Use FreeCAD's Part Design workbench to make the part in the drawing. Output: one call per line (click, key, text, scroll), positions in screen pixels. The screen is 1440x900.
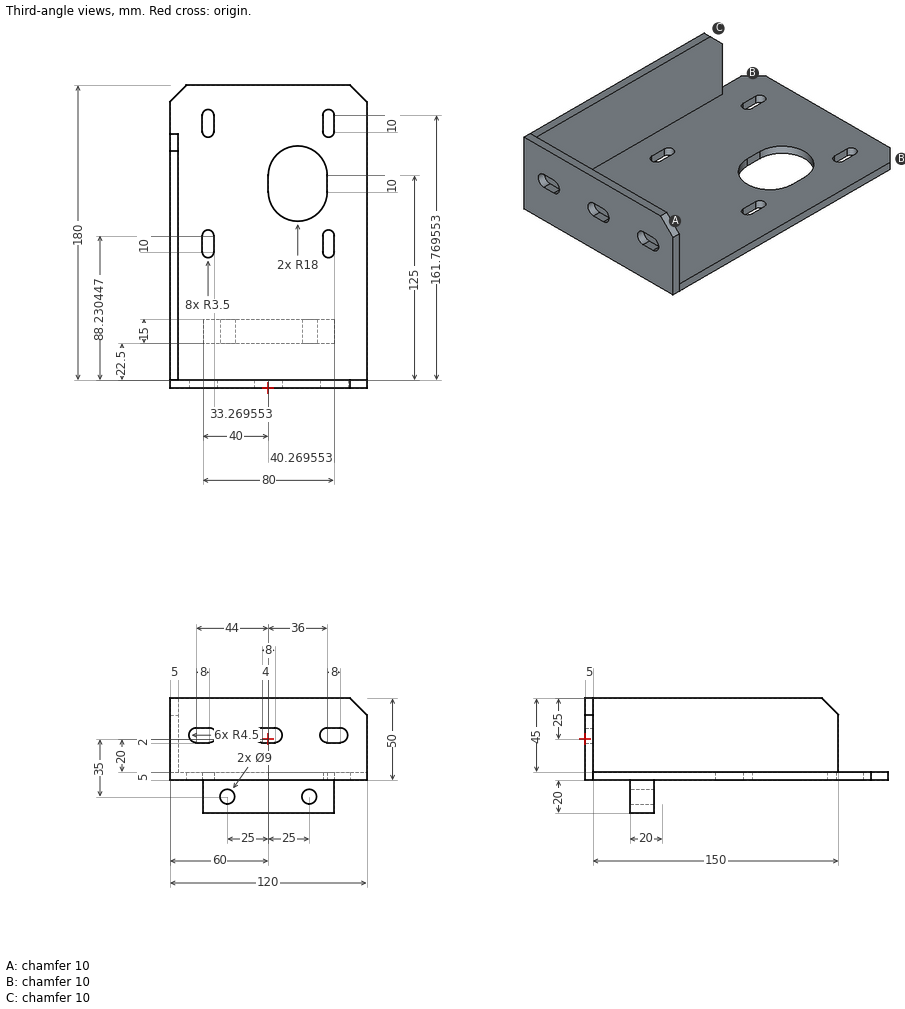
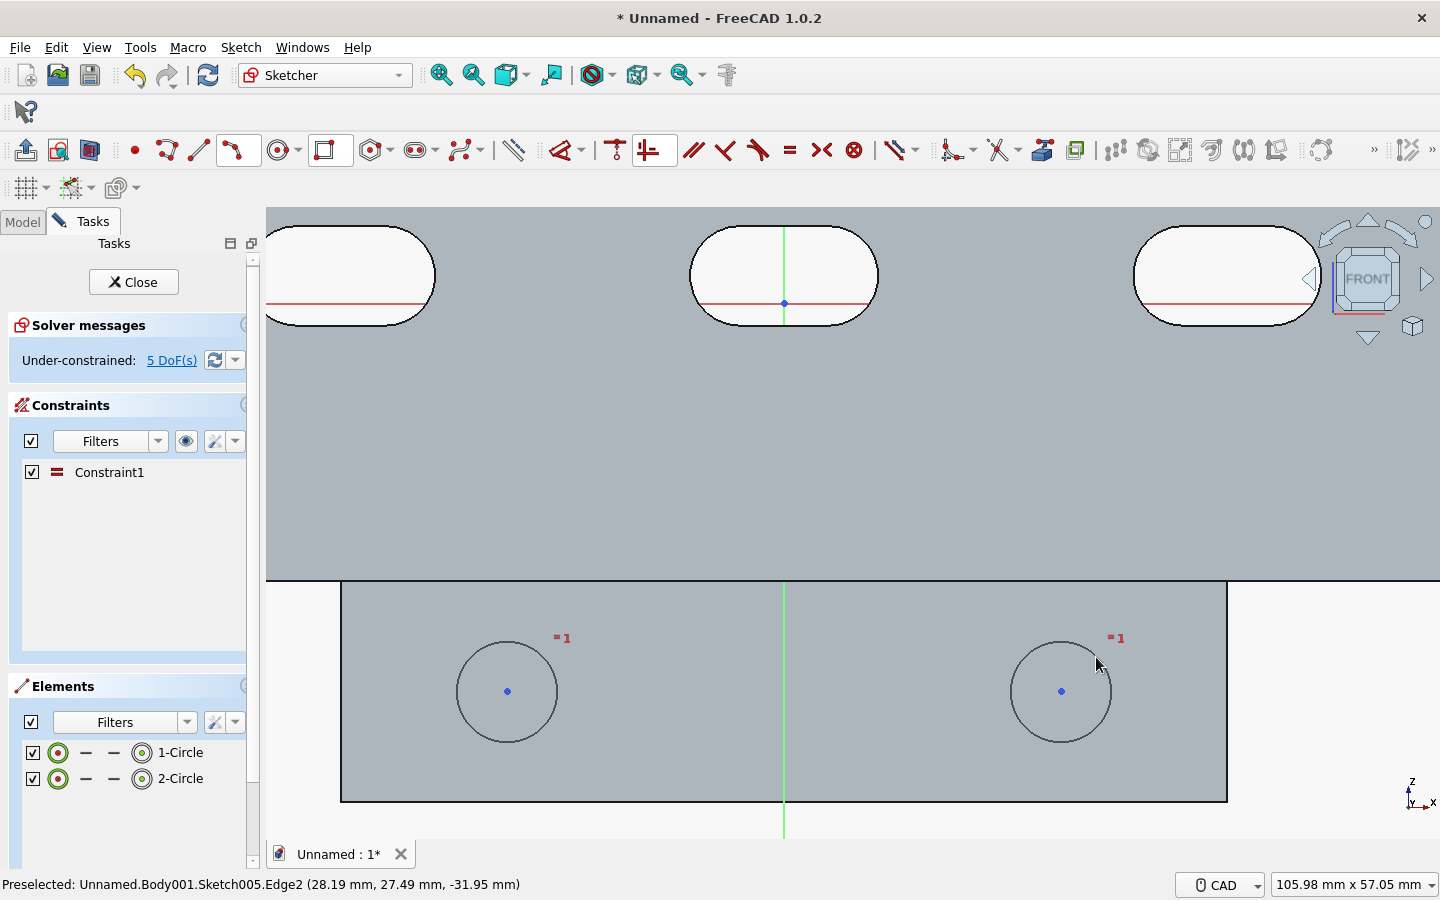
click(560, 150)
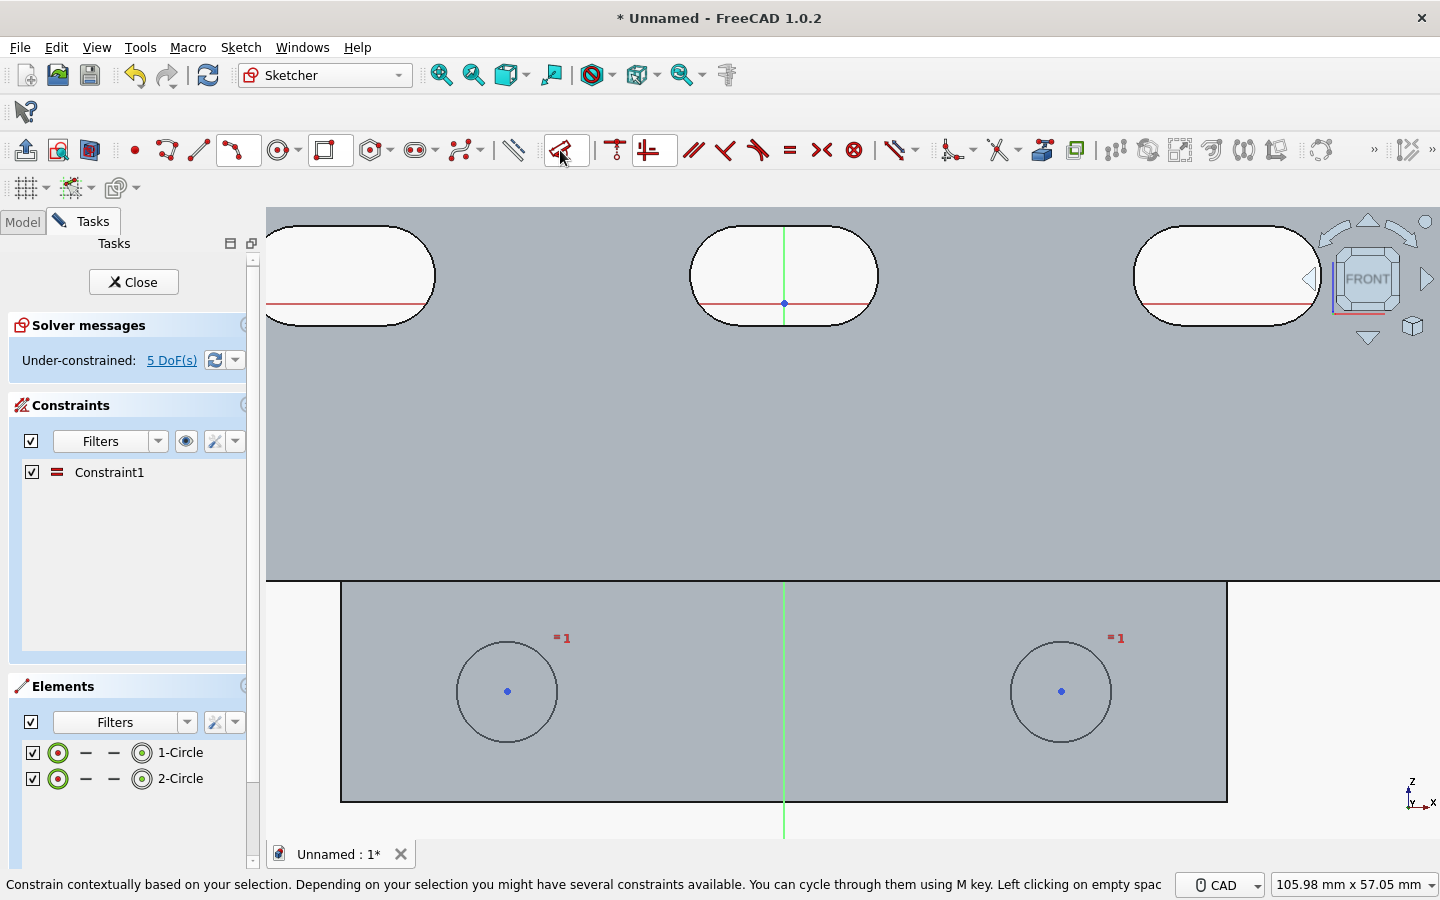
click(542, 656)
click(564, 633)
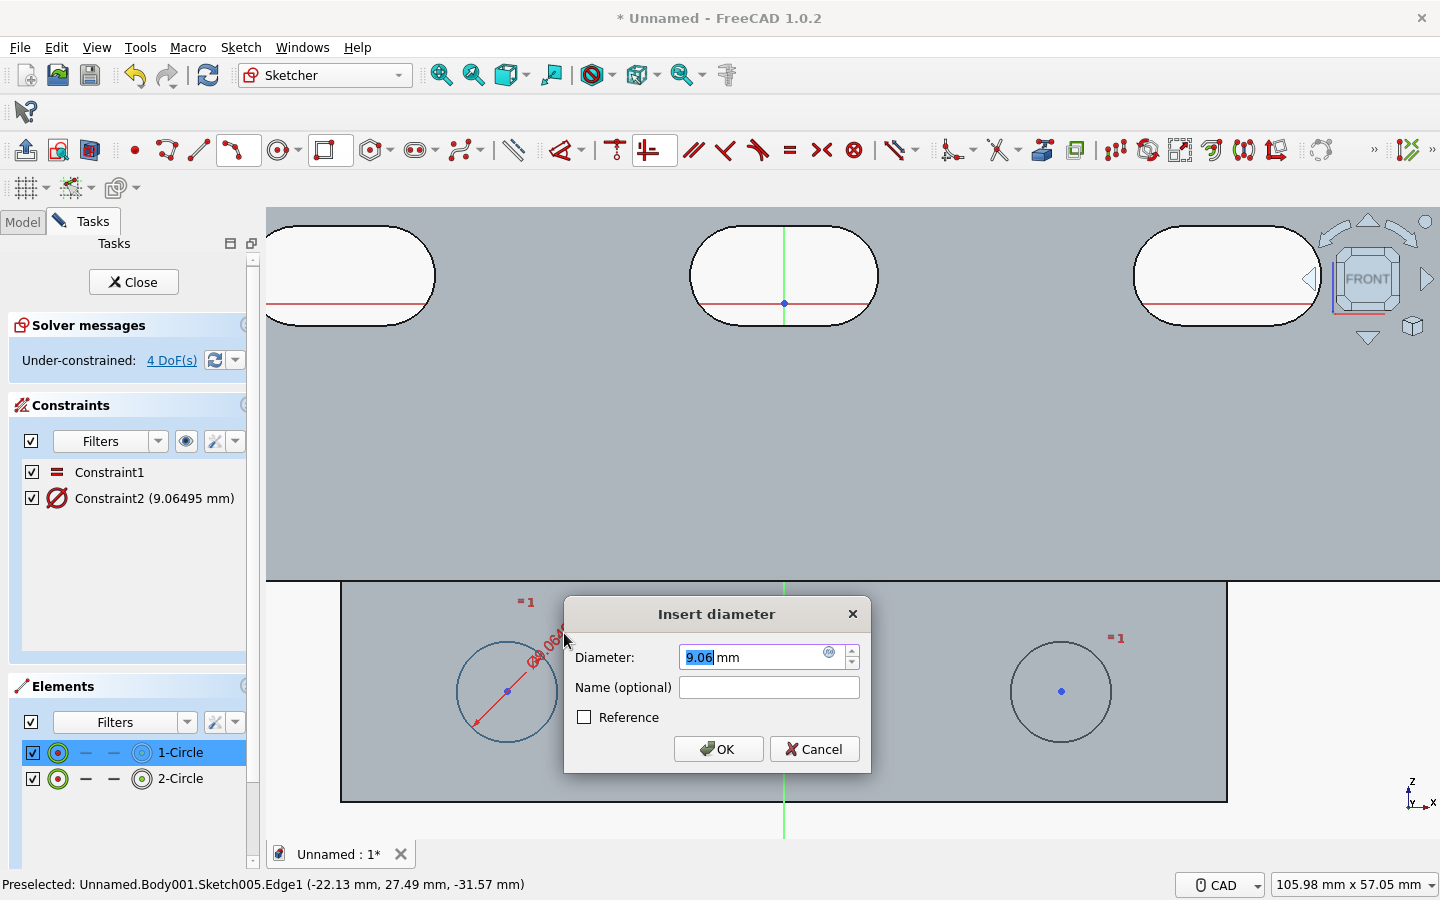
text(9)
key(Return)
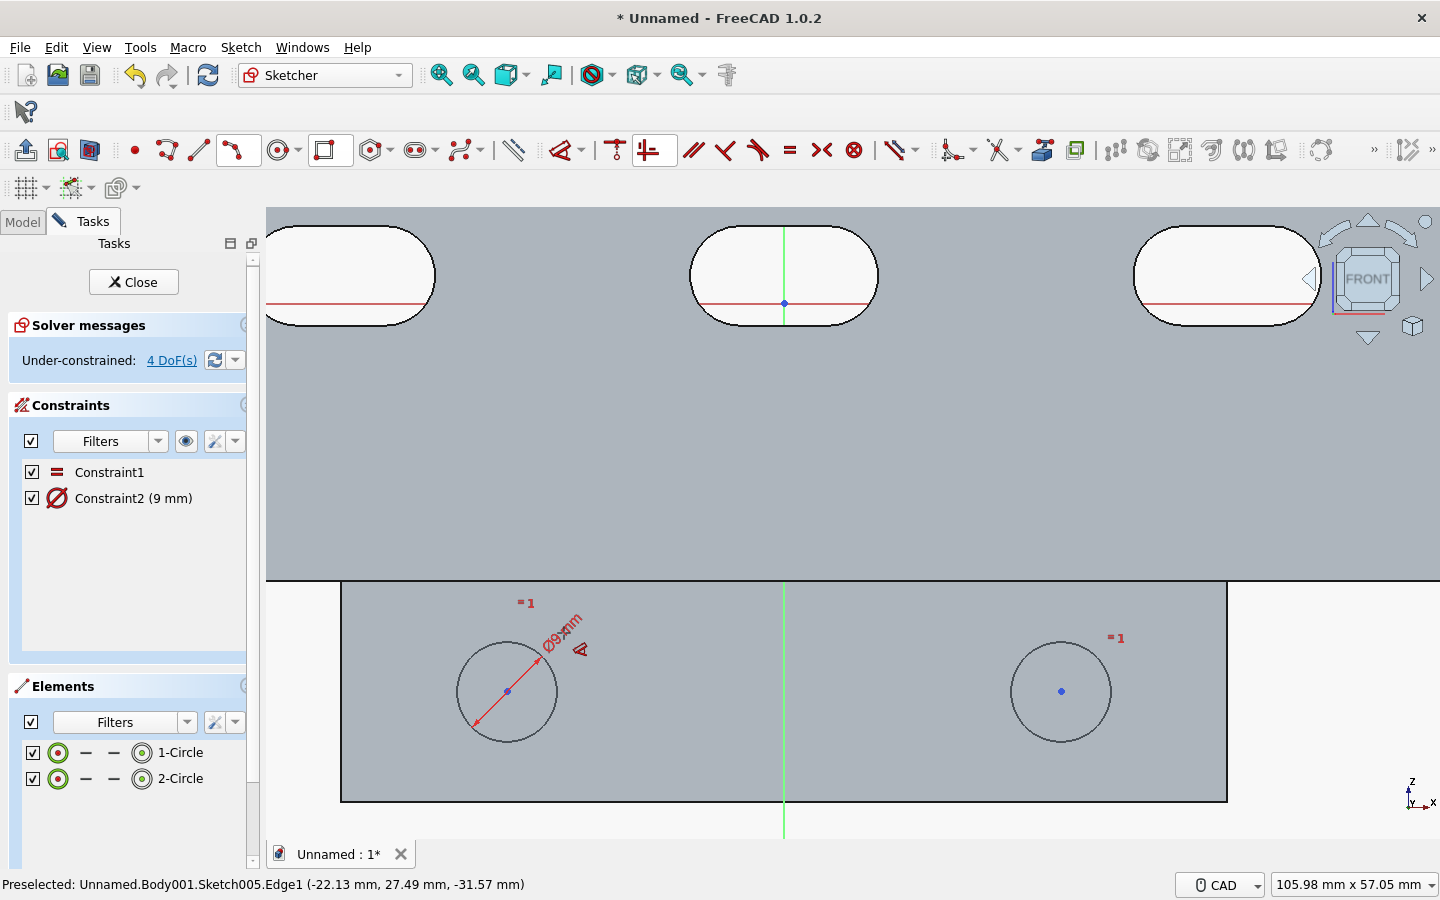
click(507, 692)
click(646, 270)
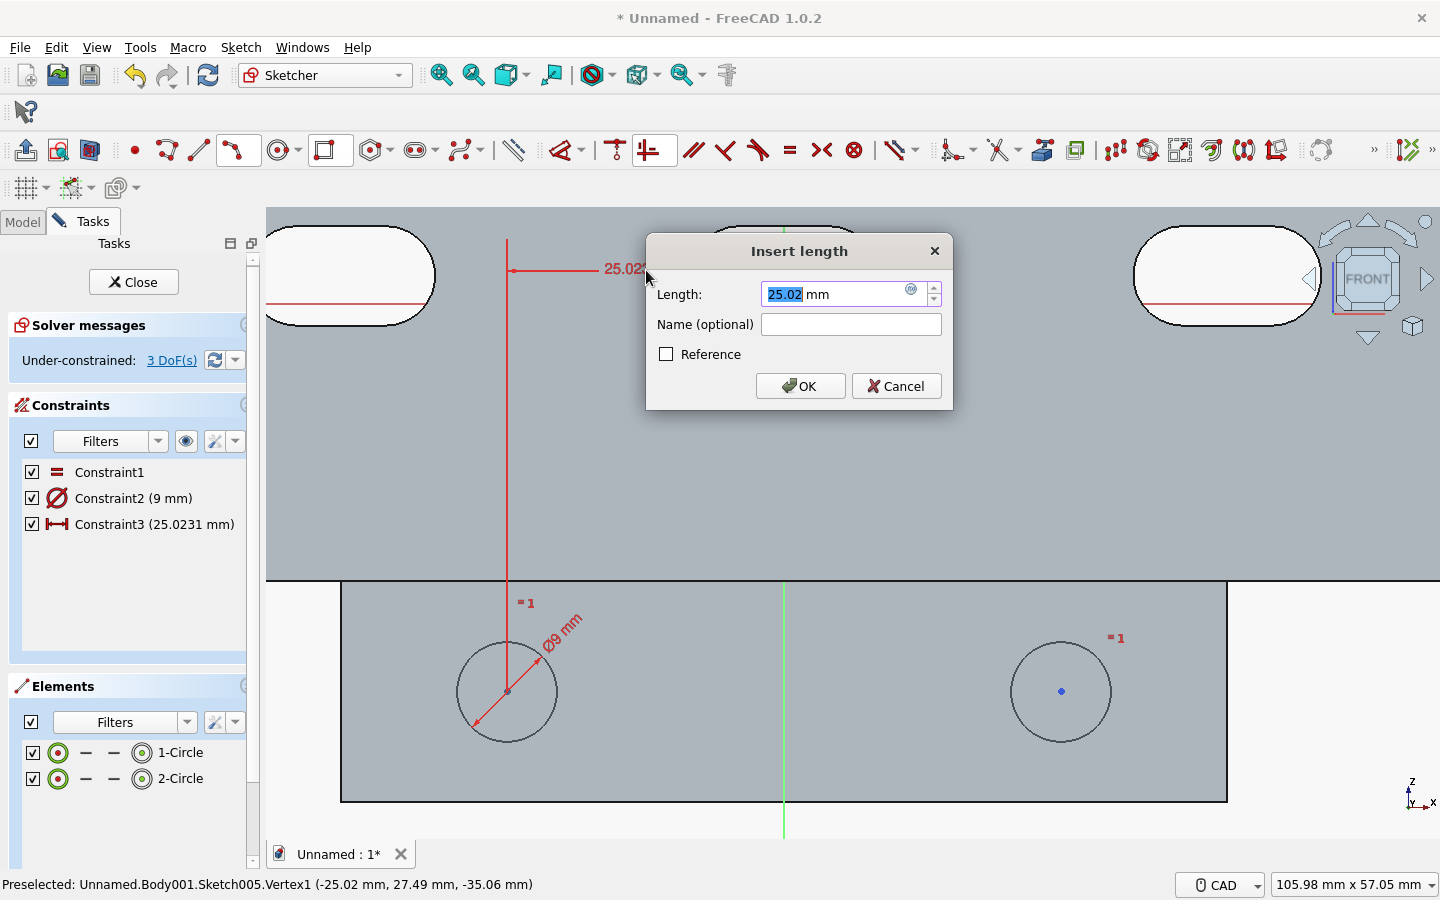
text(25)
key(Return)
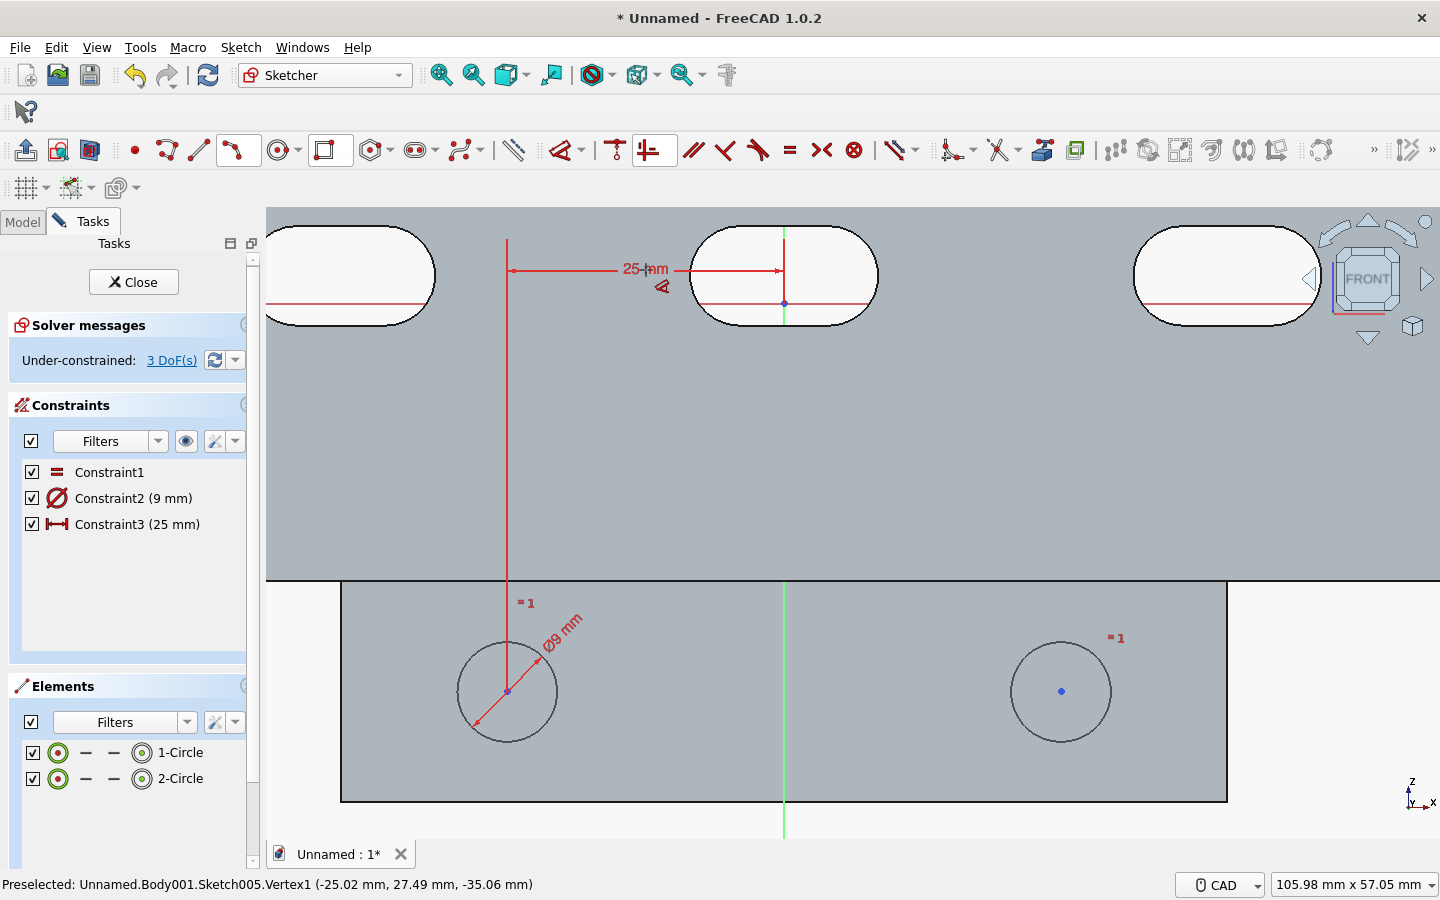
click(507, 692)
click(473, 498)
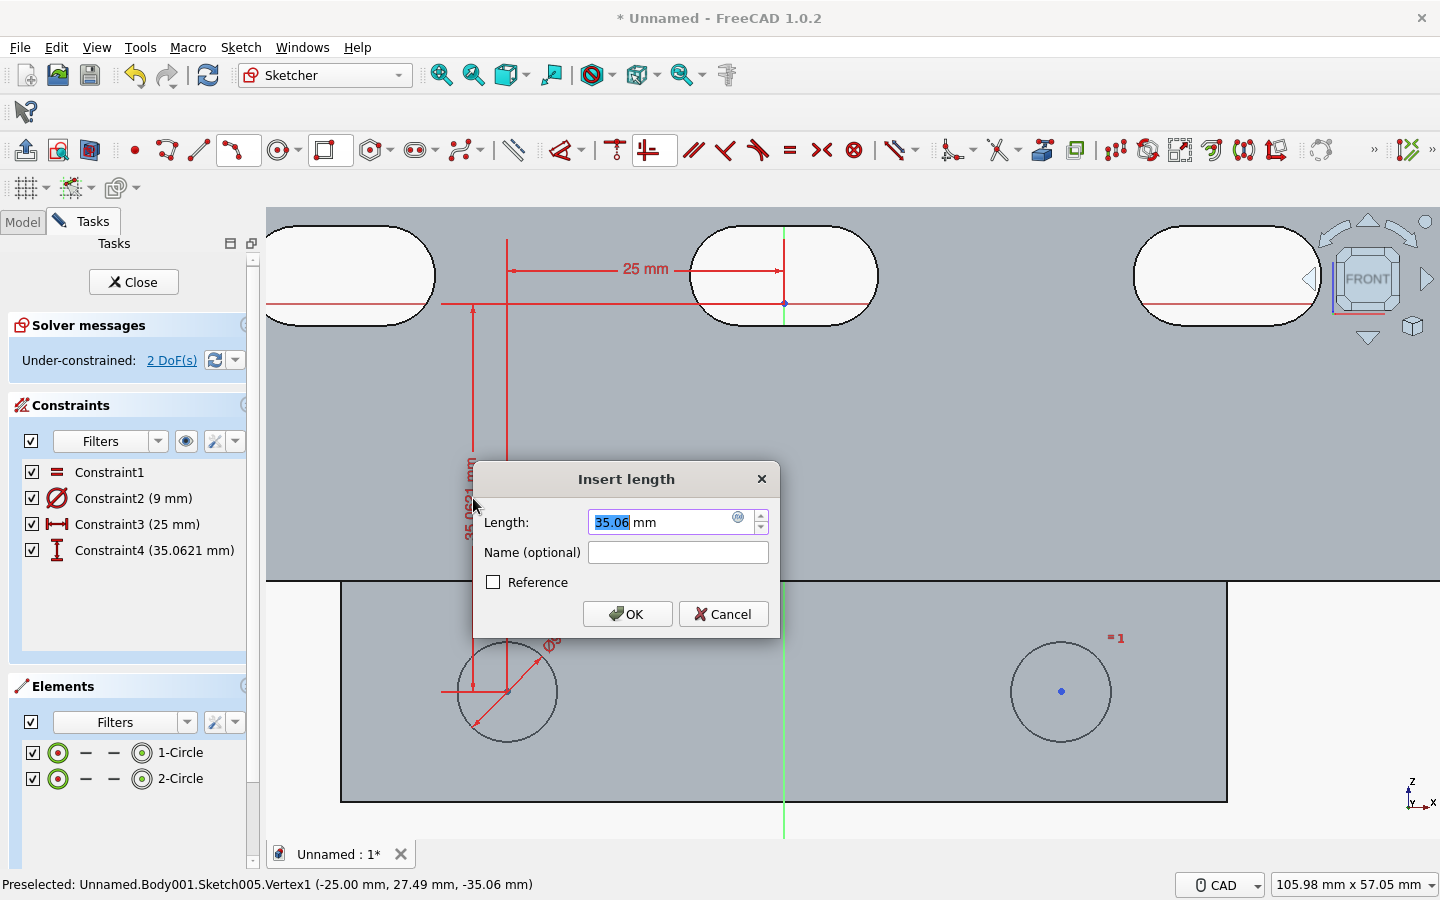
text(35)
key(Return)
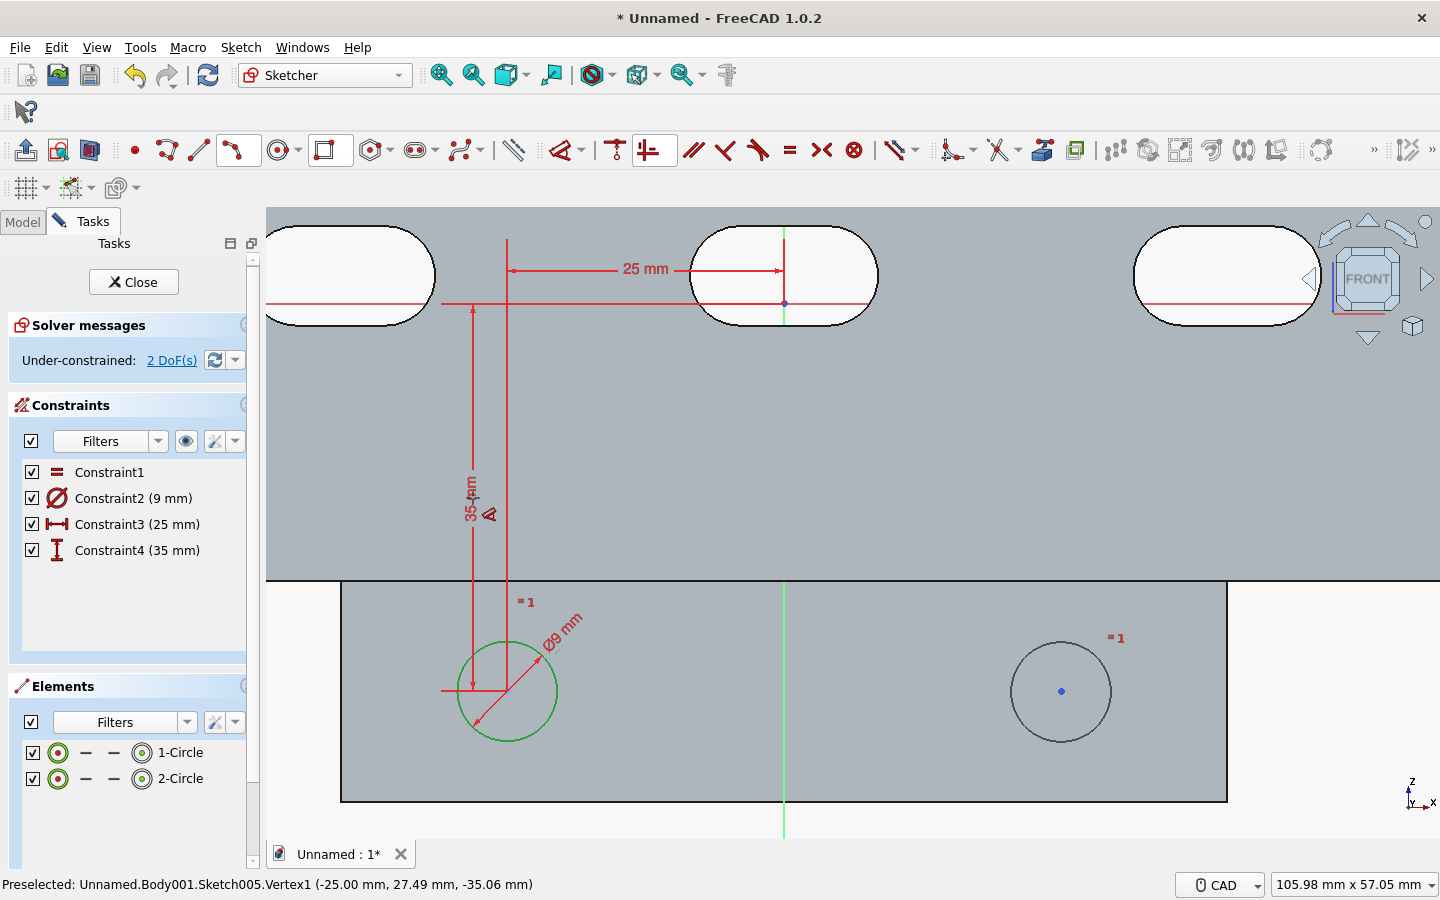
click(1061, 692)
click(923, 270)